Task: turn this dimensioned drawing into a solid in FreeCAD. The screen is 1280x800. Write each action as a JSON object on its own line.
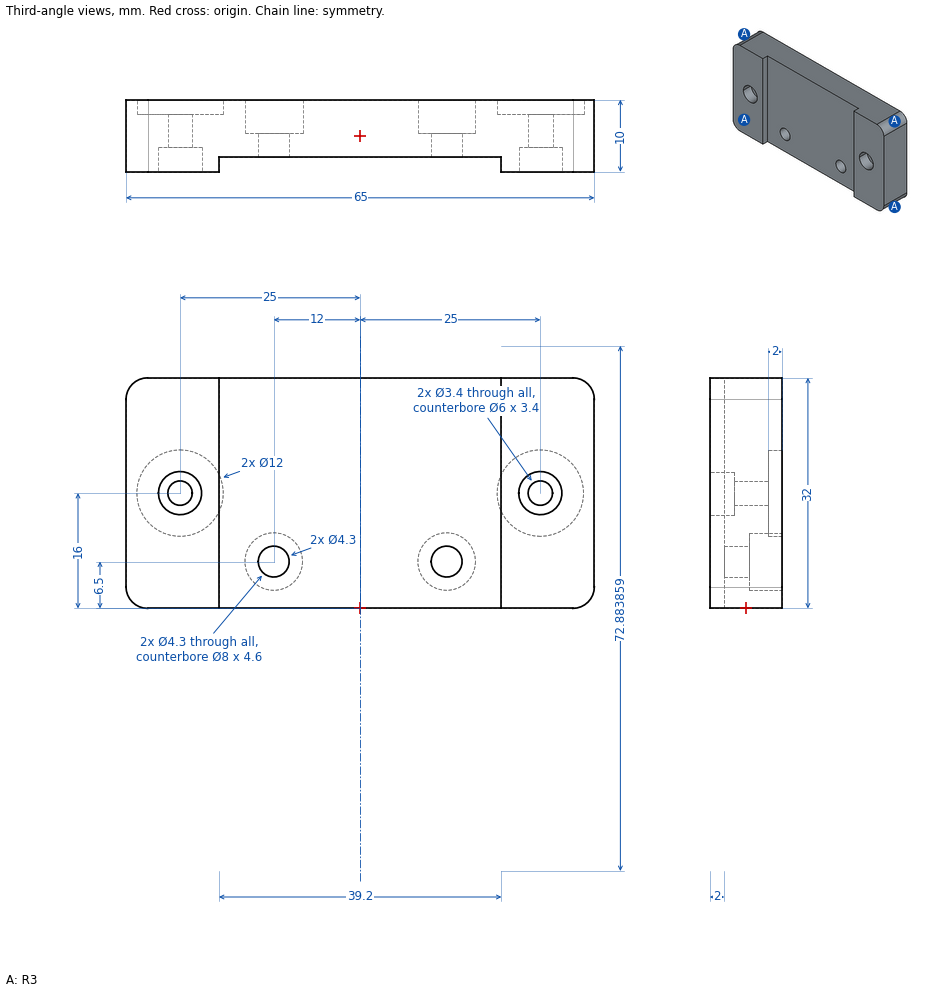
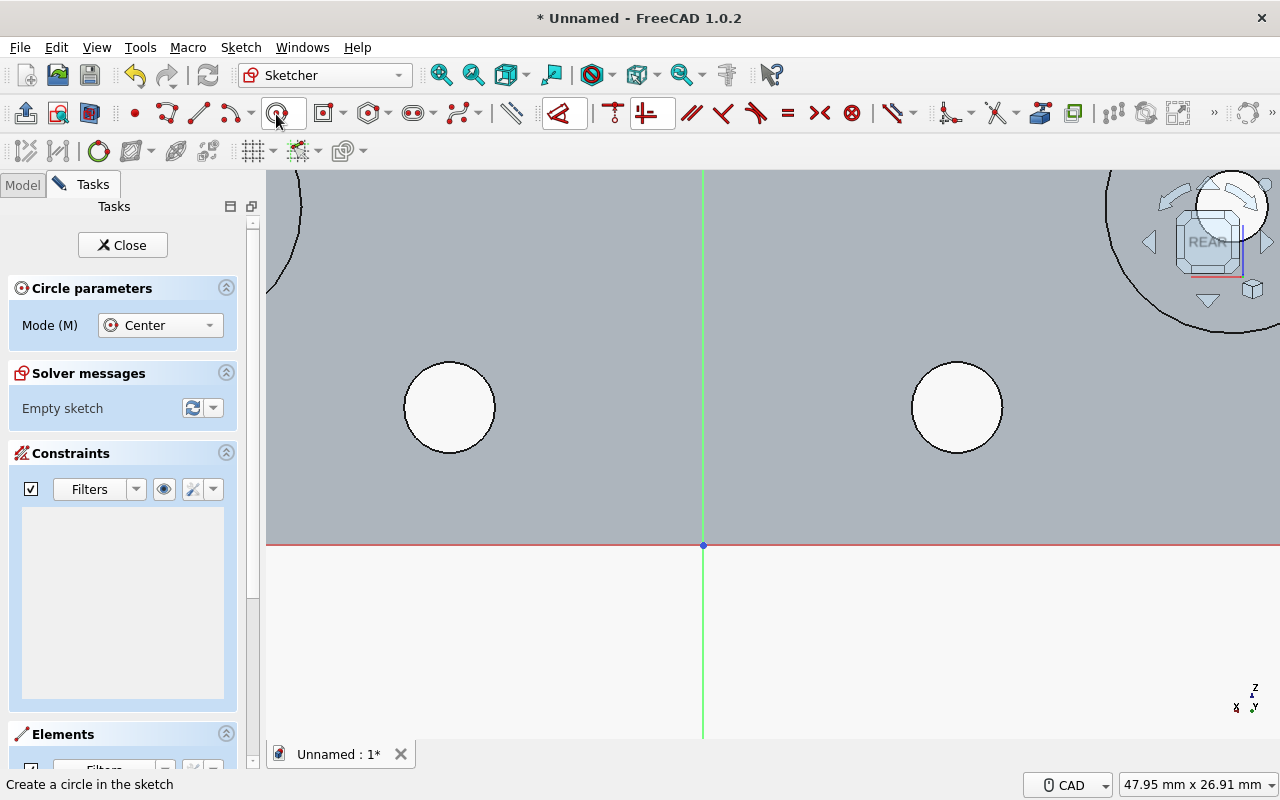
{"action": "left_click", "coordinate": [957, 408]}
{"action": "left_click", "coordinate": [989, 375]}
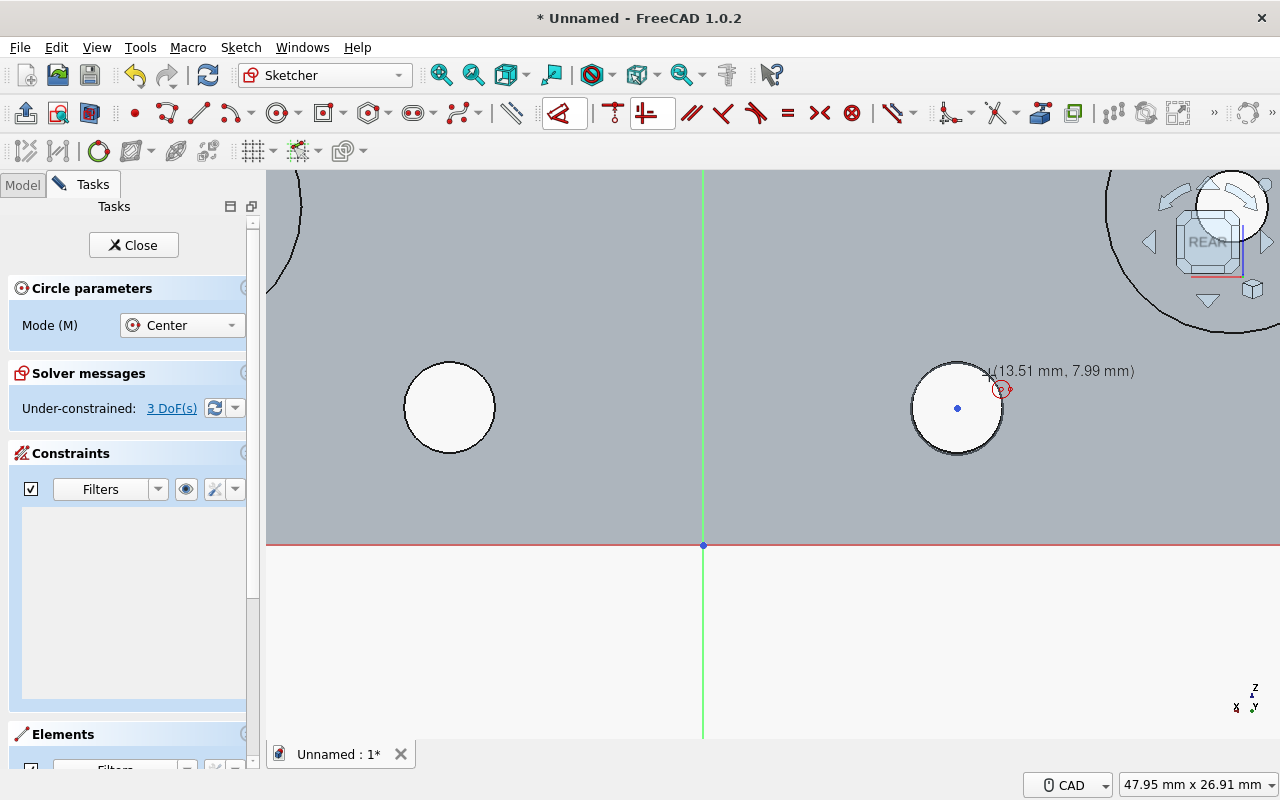
{"action": "left_click", "coordinate": [450, 408]}
{"action": "left_click", "coordinate": [482, 375]}
{"action": "key", "text": "Escape"}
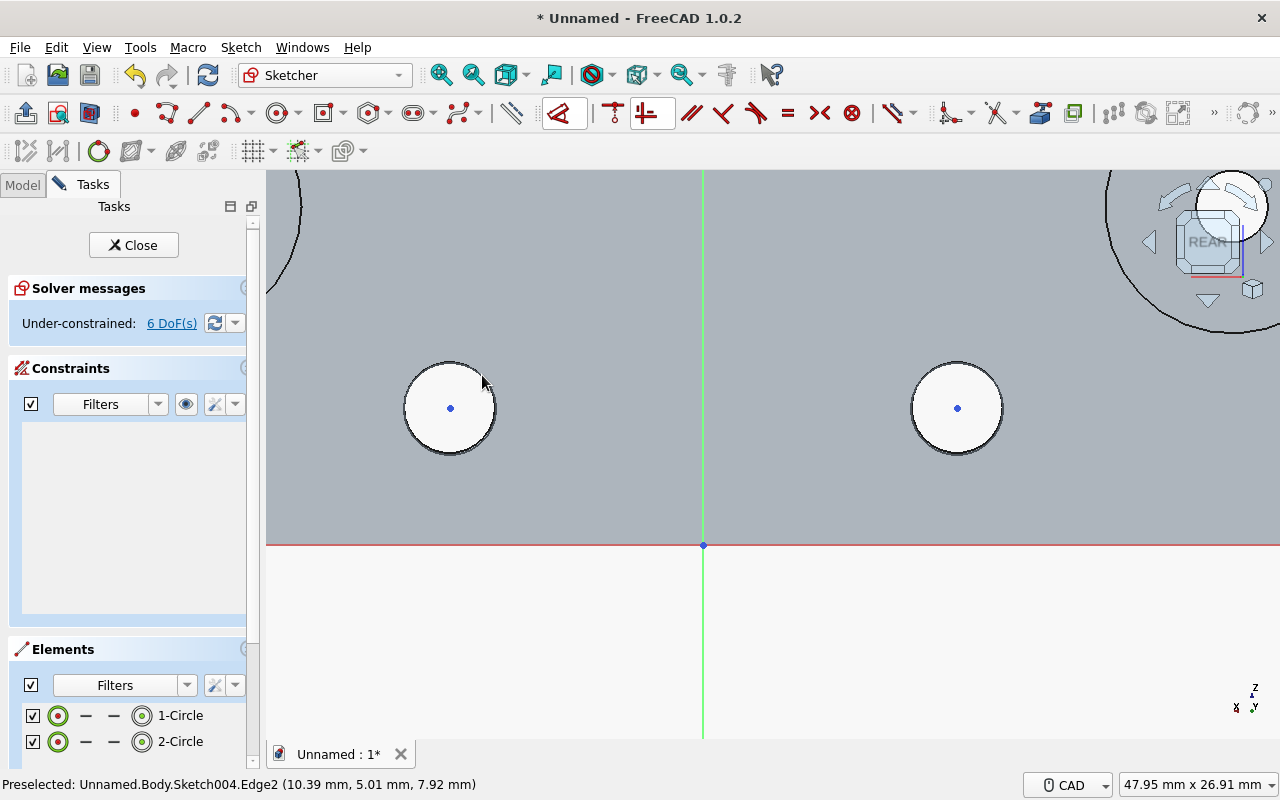
{"action": "left_click", "coordinate": [989, 376]}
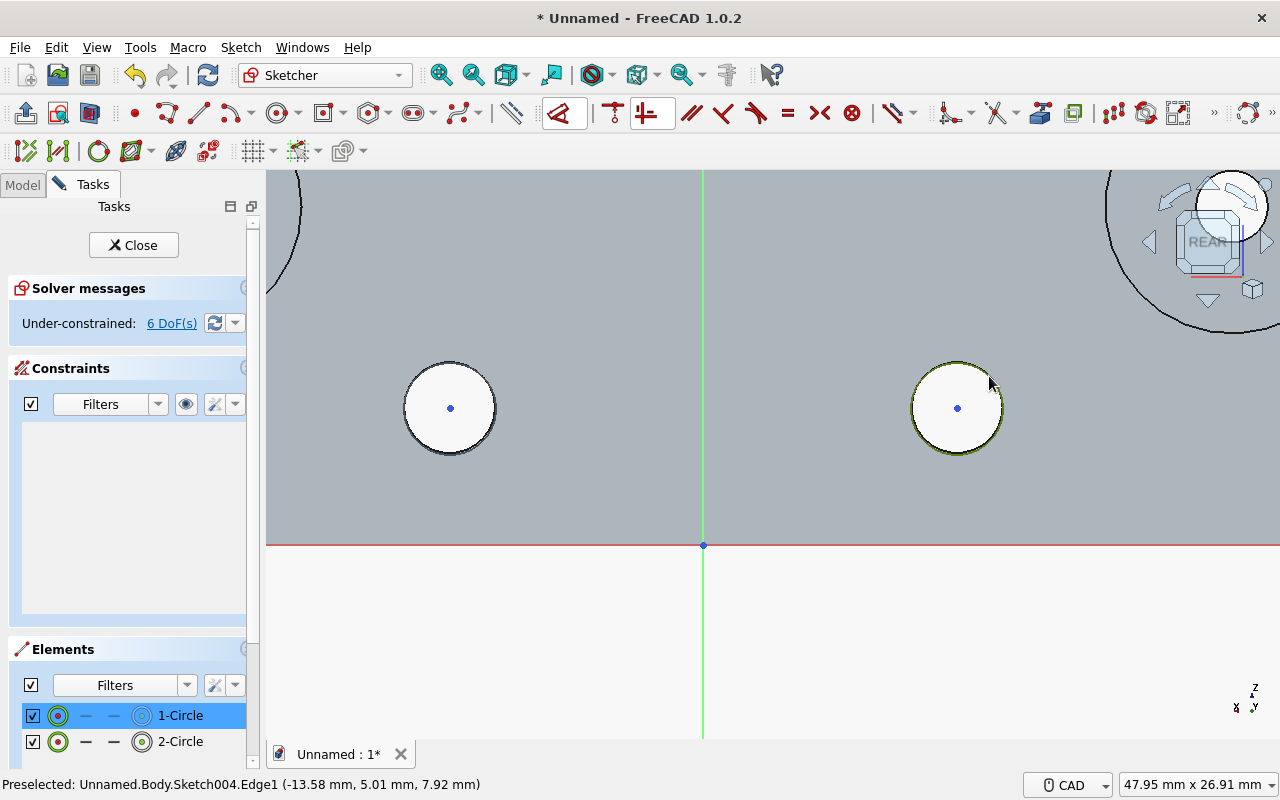
{"action": "left_click", "coordinate": [482, 376]}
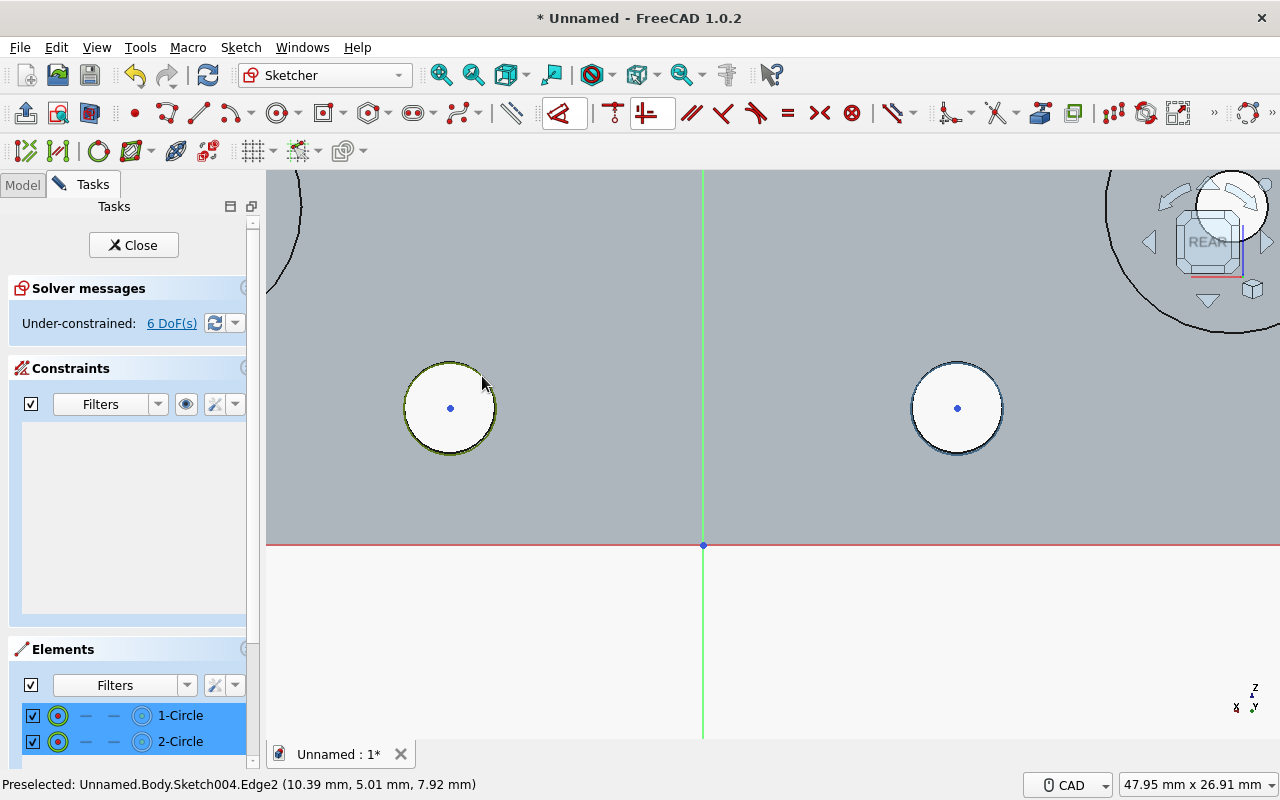
{"action": "left_click", "coordinate": [788, 114]}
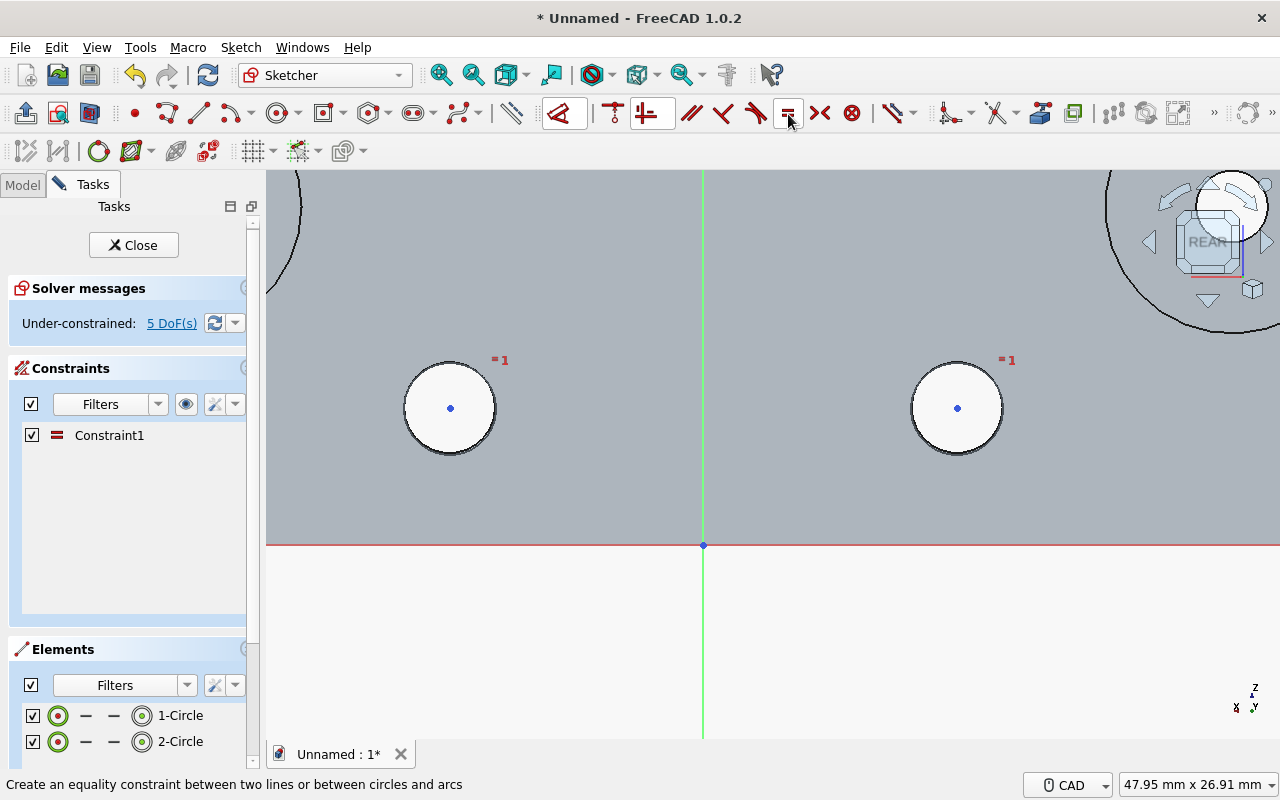
{"action": "left_click", "coordinate": [957, 409]}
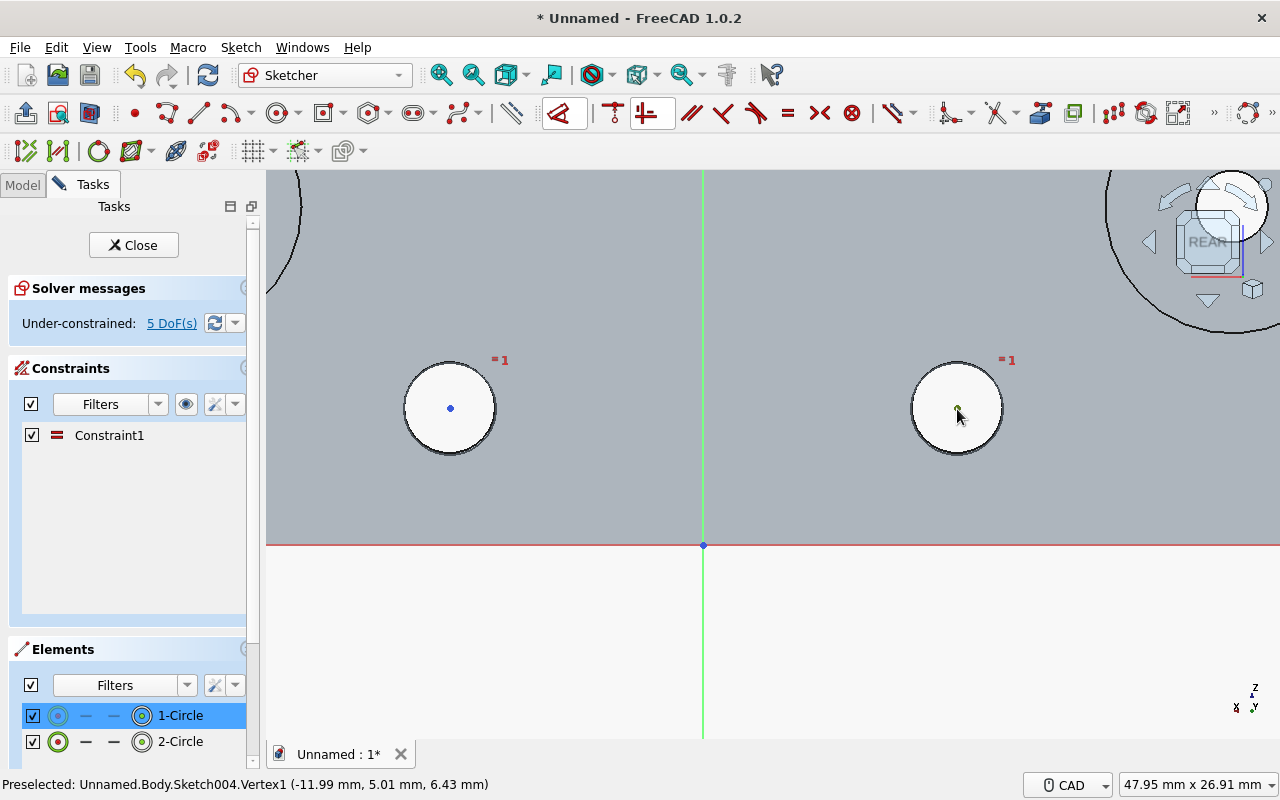
{"action": "left_click", "coordinate": [450, 409]}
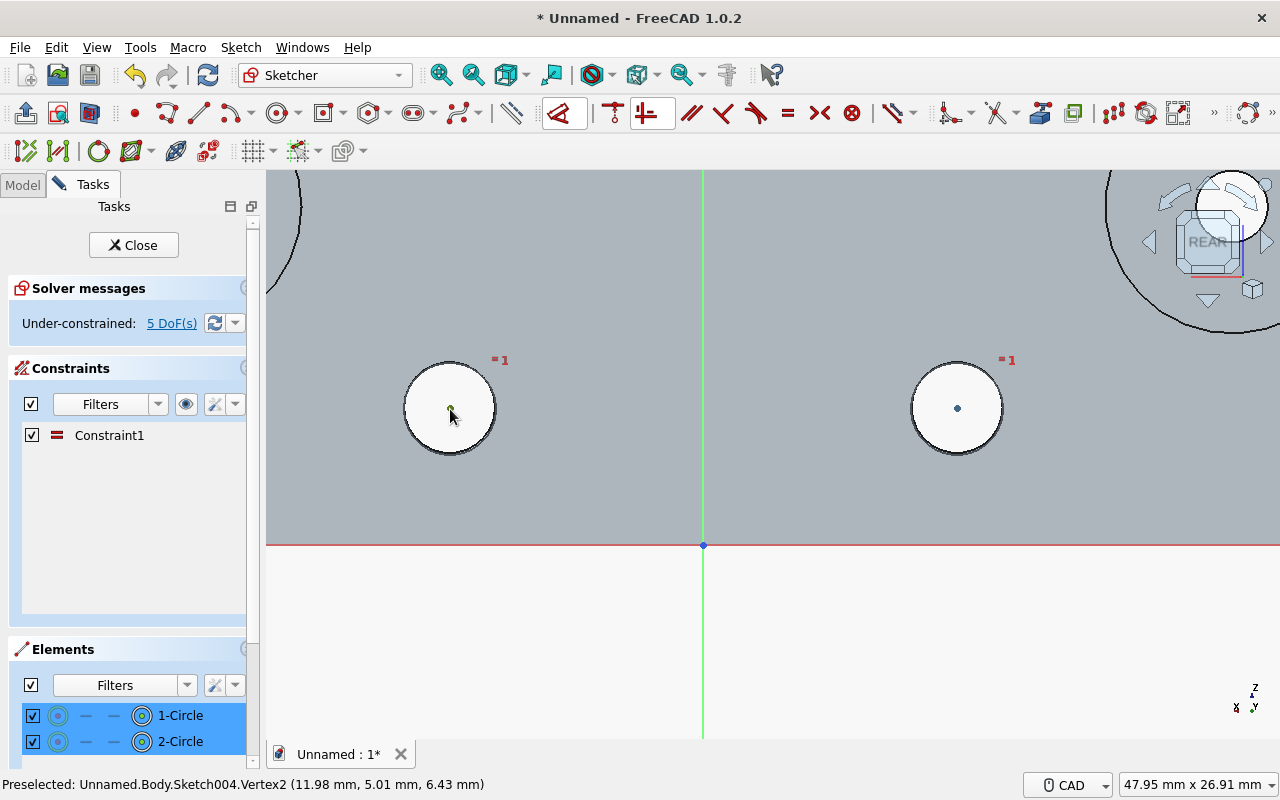
{"action": "left_click", "coordinate": [703, 674]}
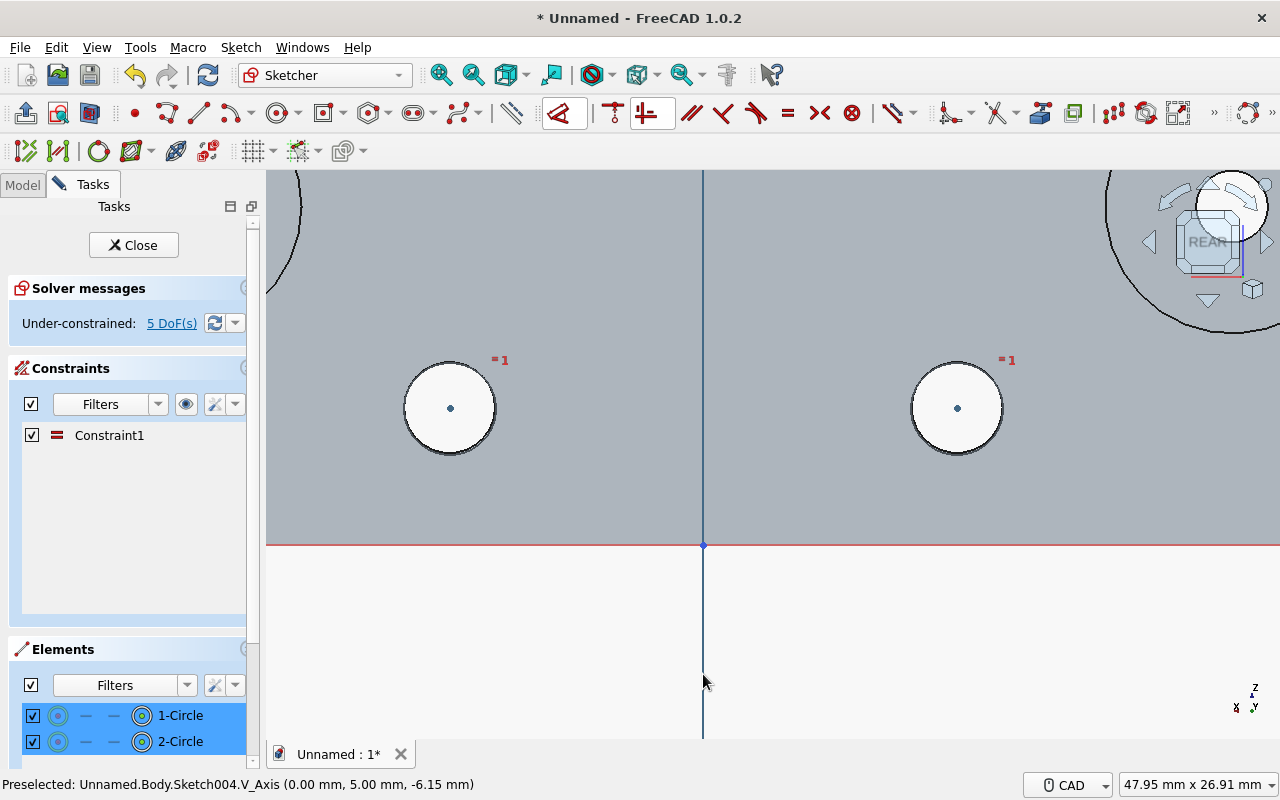
{"action": "left_click", "coordinate": [820, 114]}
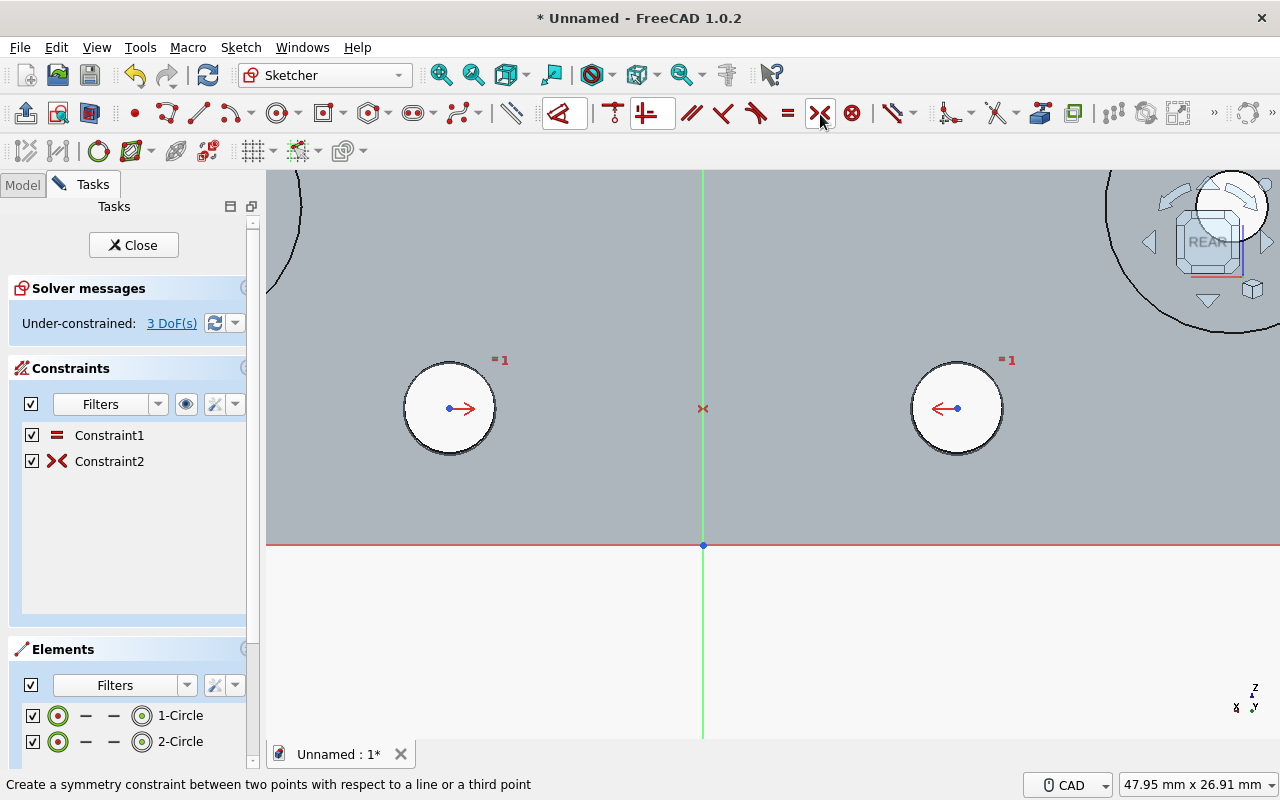
{"action": "left_click", "coordinate": [989, 376]}